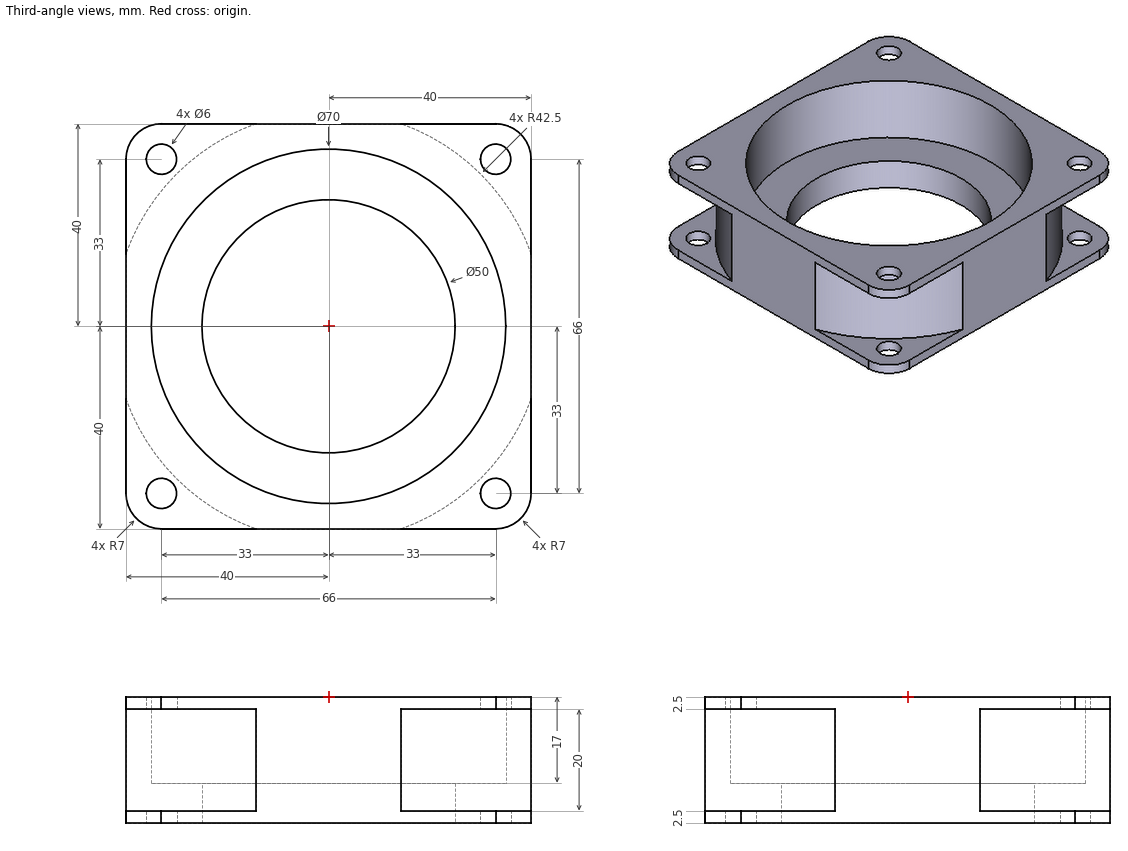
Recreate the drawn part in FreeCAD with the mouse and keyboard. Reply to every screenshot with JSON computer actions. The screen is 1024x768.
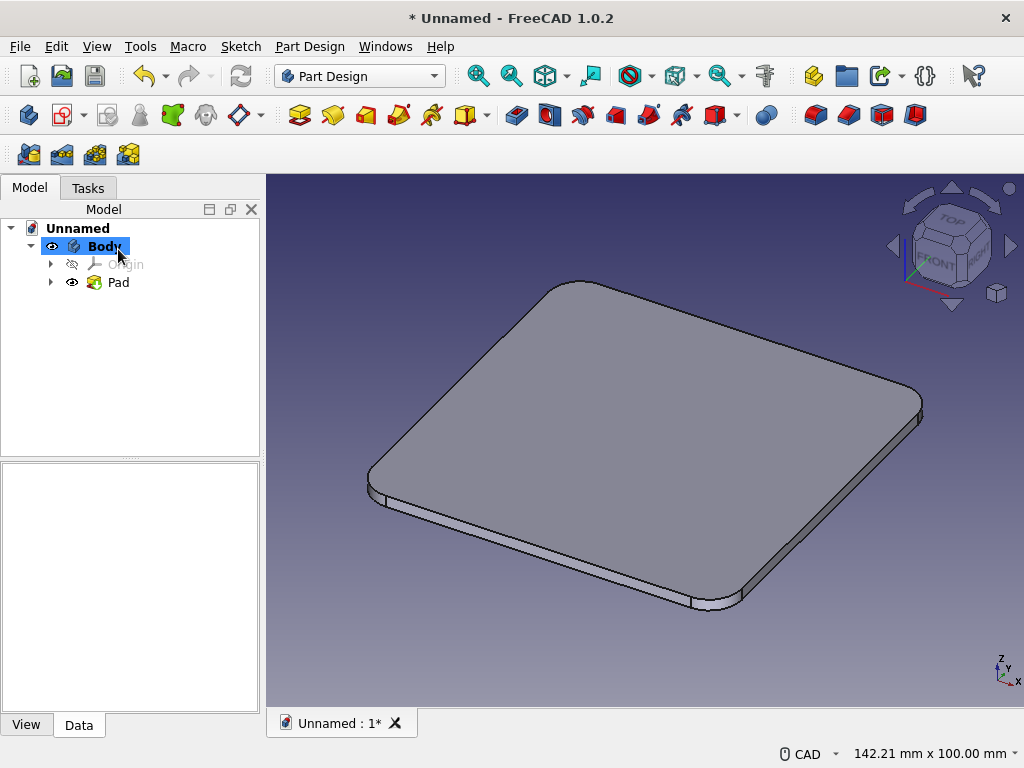
{"action": "key", "text": "5"}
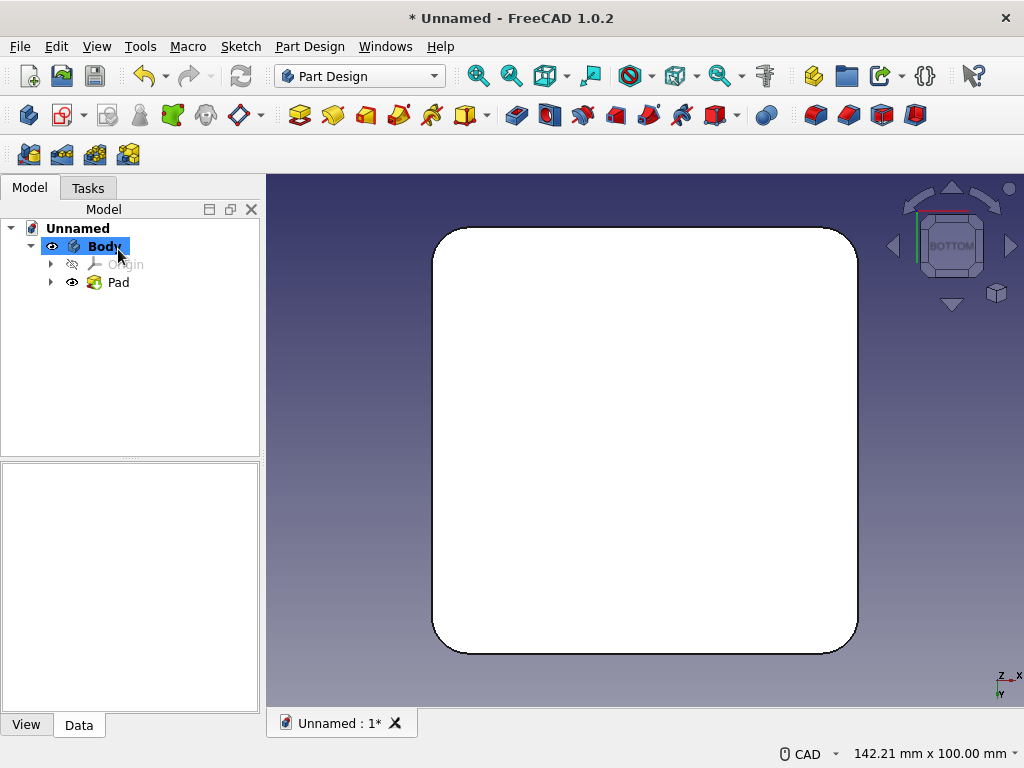
{"action": "left_click", "coordinate": [645, 439]}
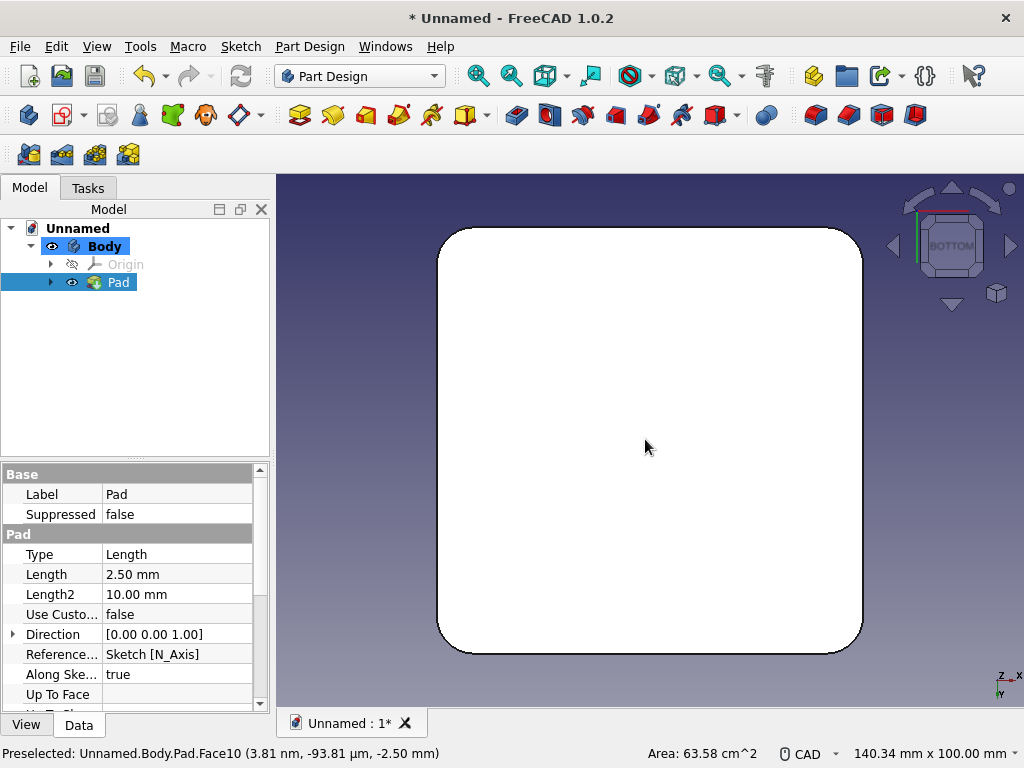
{"action": "left_click", "coordinate": [62, 116]}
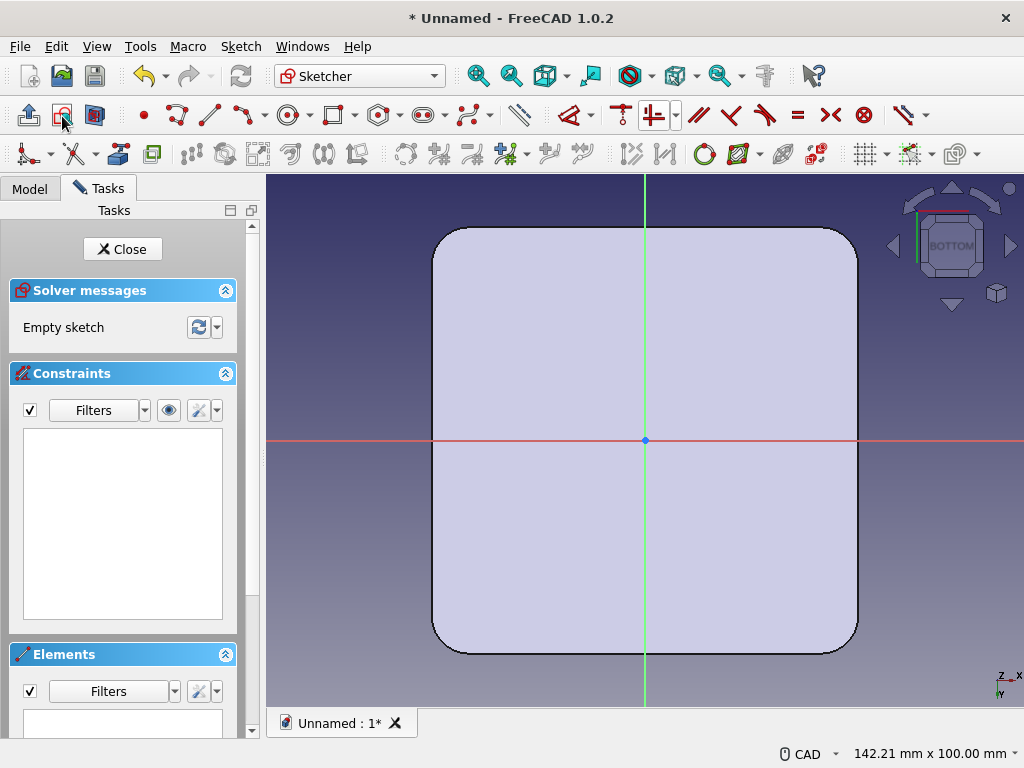
{"action": "scroll", "coordinate": [294, 440], "scroll_direction": "down", "scroll_amount": 1}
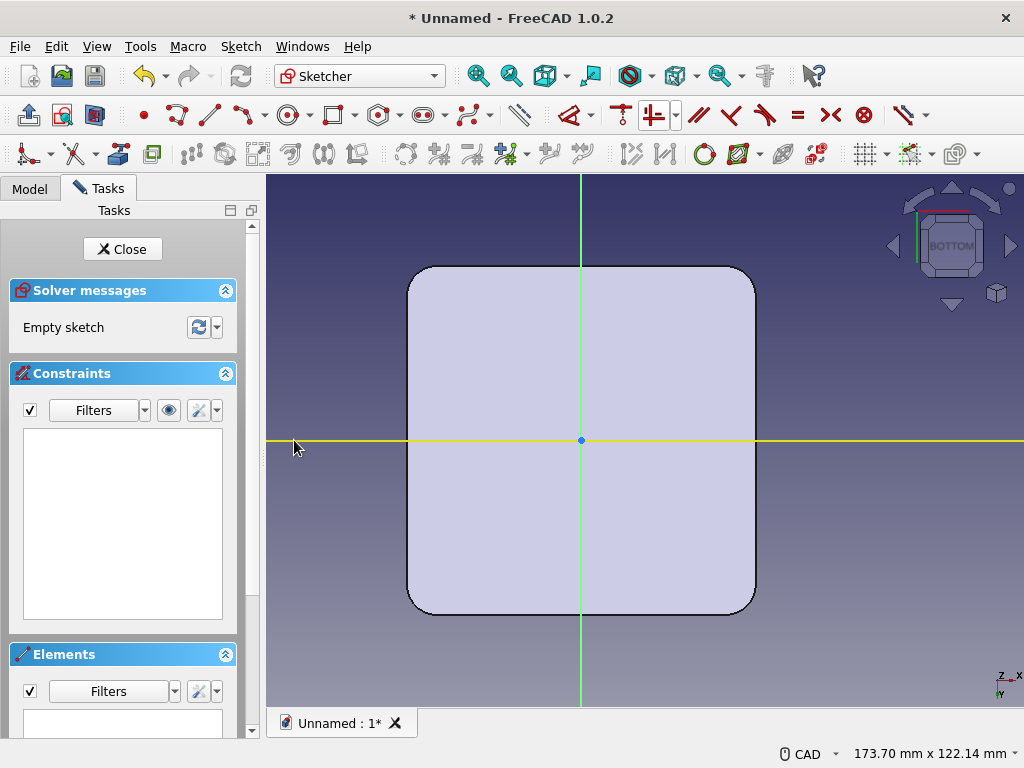
{"action": "left_click", "coordinate": [210, 116]}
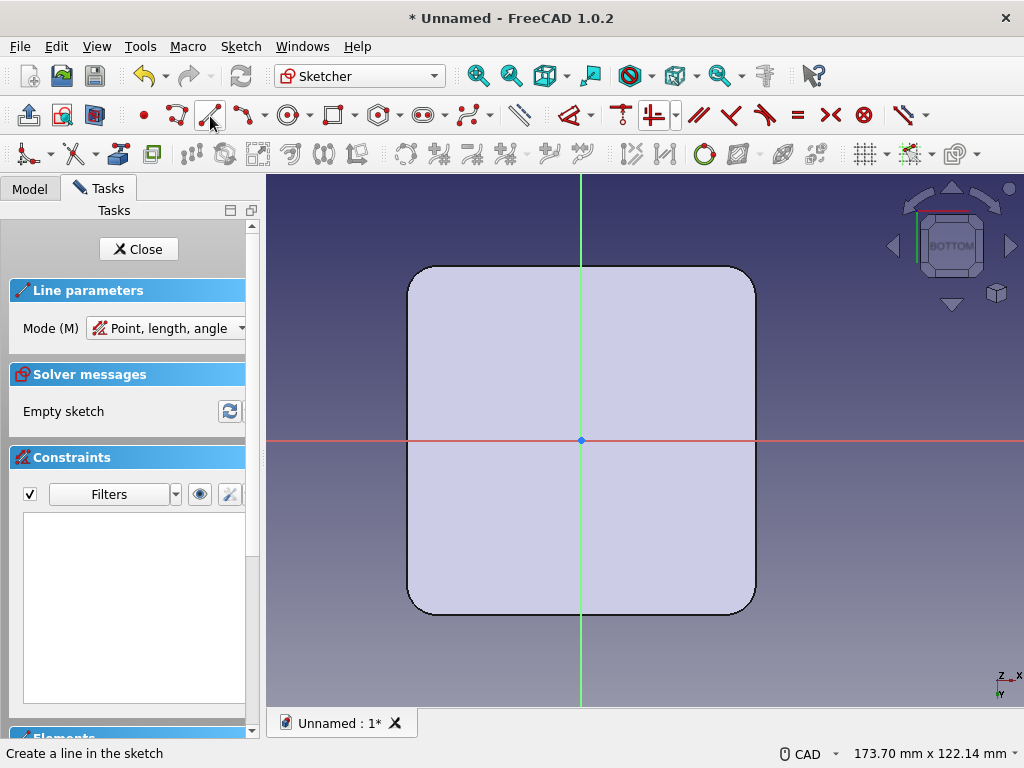
{"action": "left_click", "coordinate": [519, 615]}
{"action": "left_click", "coordinate": [644, 615]}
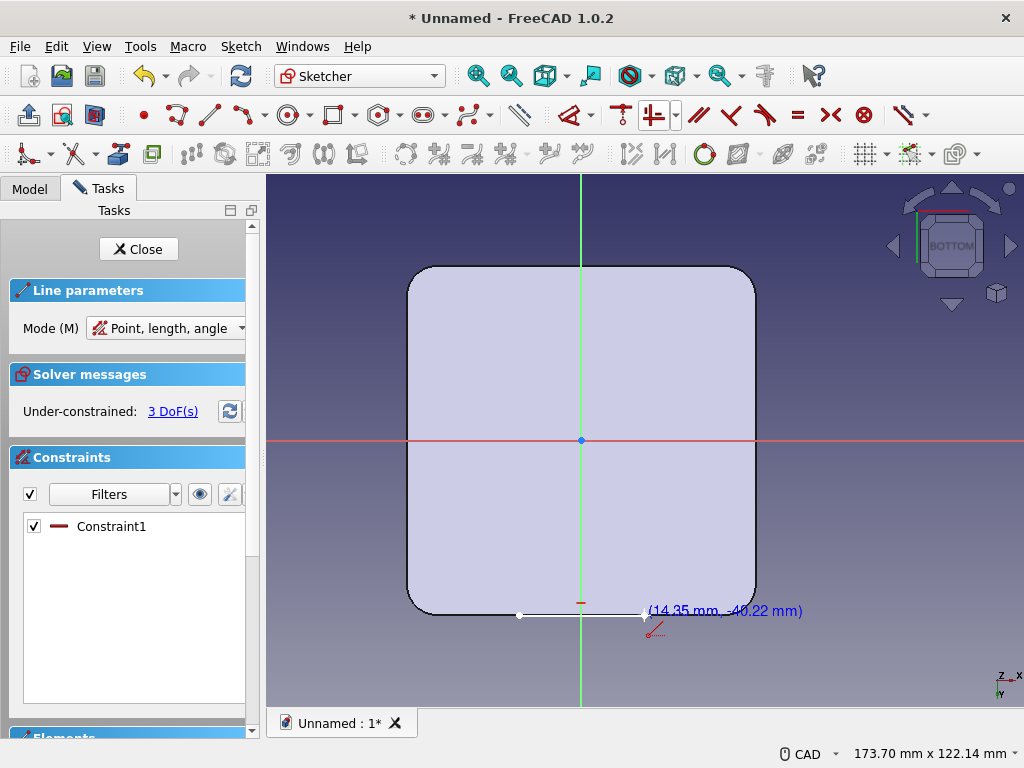
{"action": "left_click", "coordinate": [756, 503]}
{"action": "left_click", "coordinate": [756, 378]}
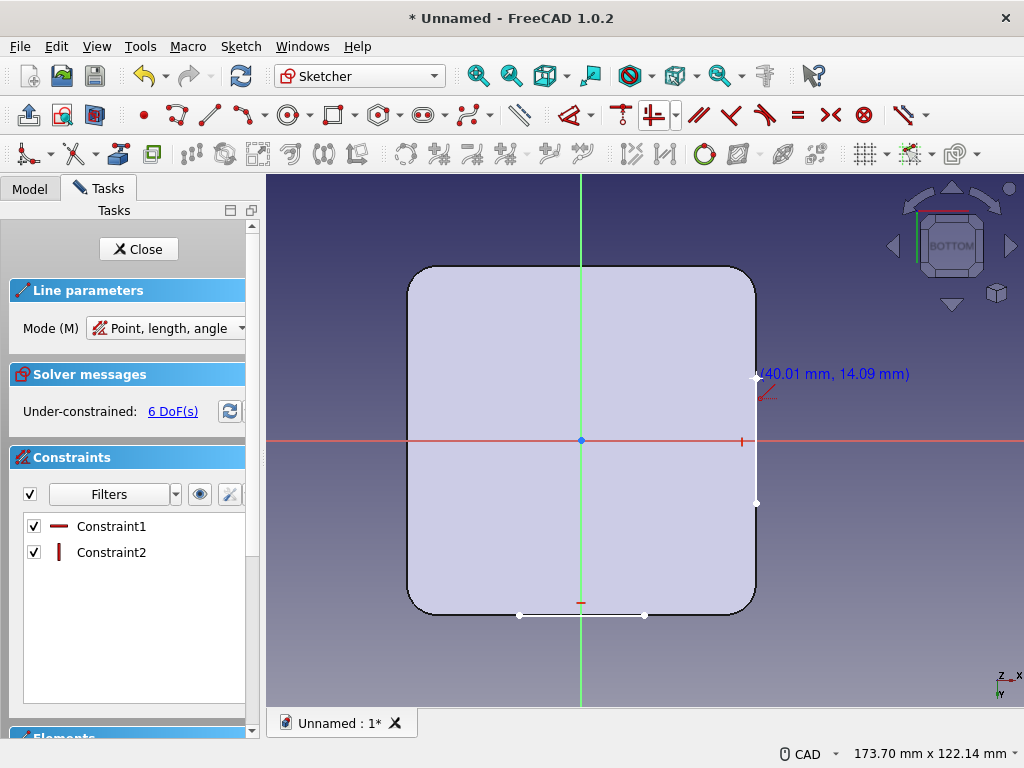
{"action": "left_click", "coordinate": [644, 266]}
{"action": "left_click", "coordinate": [519, 266]}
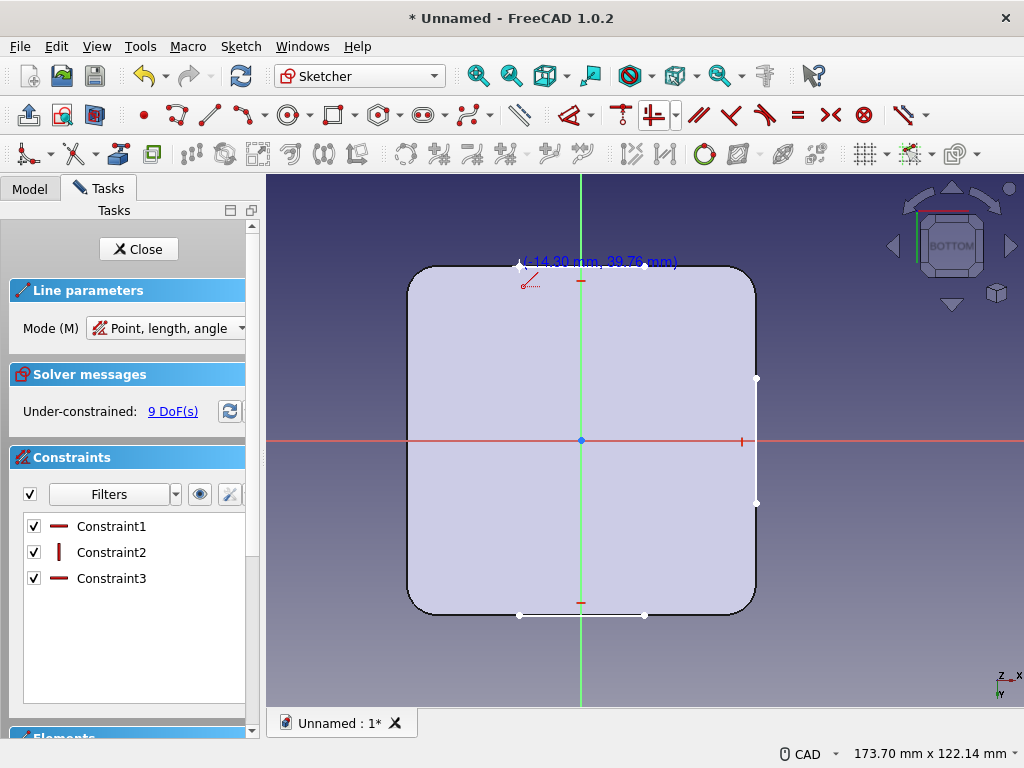
{"action": "left_click", "coordinate": [407, 378]}
{"action": "left_click", "coordinate": [407, 503]}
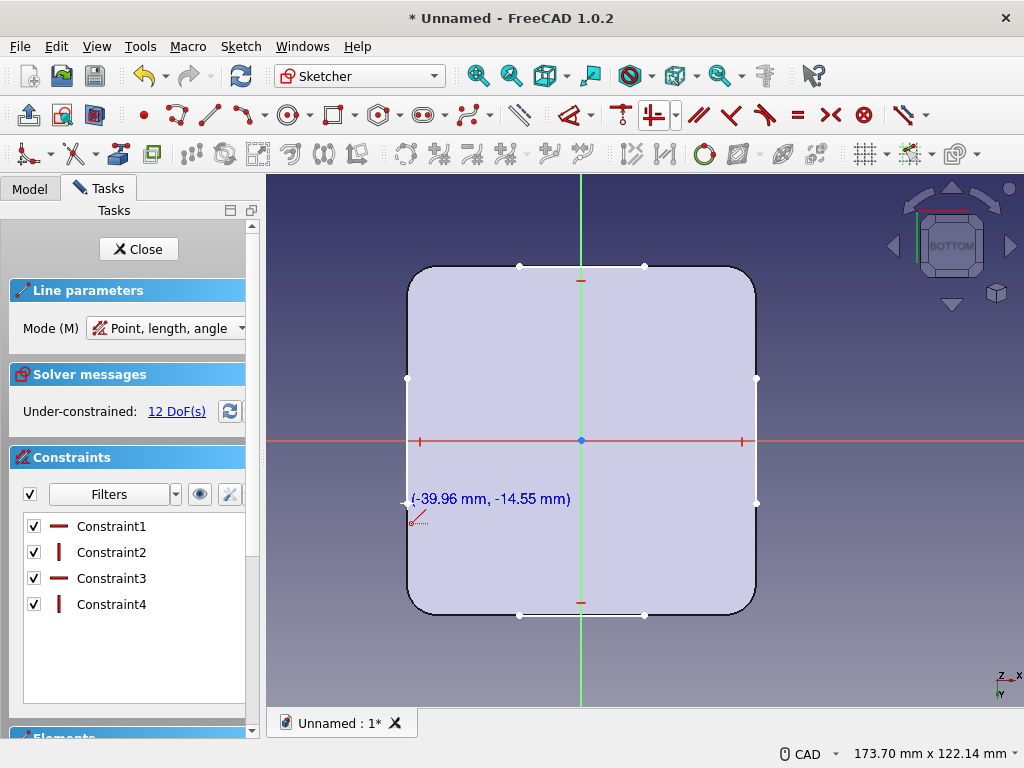
{"action": "left_click", "coordinate": [242, 116]}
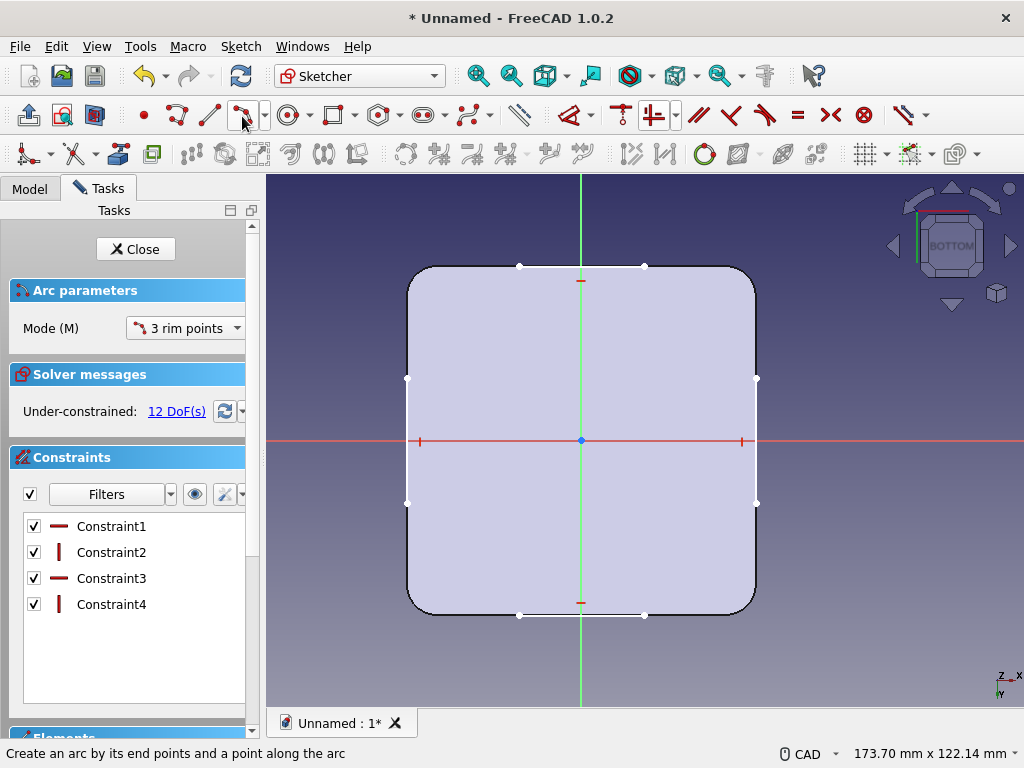
{"action": "left_click", "coordinate": [644, 616]}
{"action": "left_click", "coordinate": [756, 504]}
{"action": "left_click", "coordinate": [713, 572]}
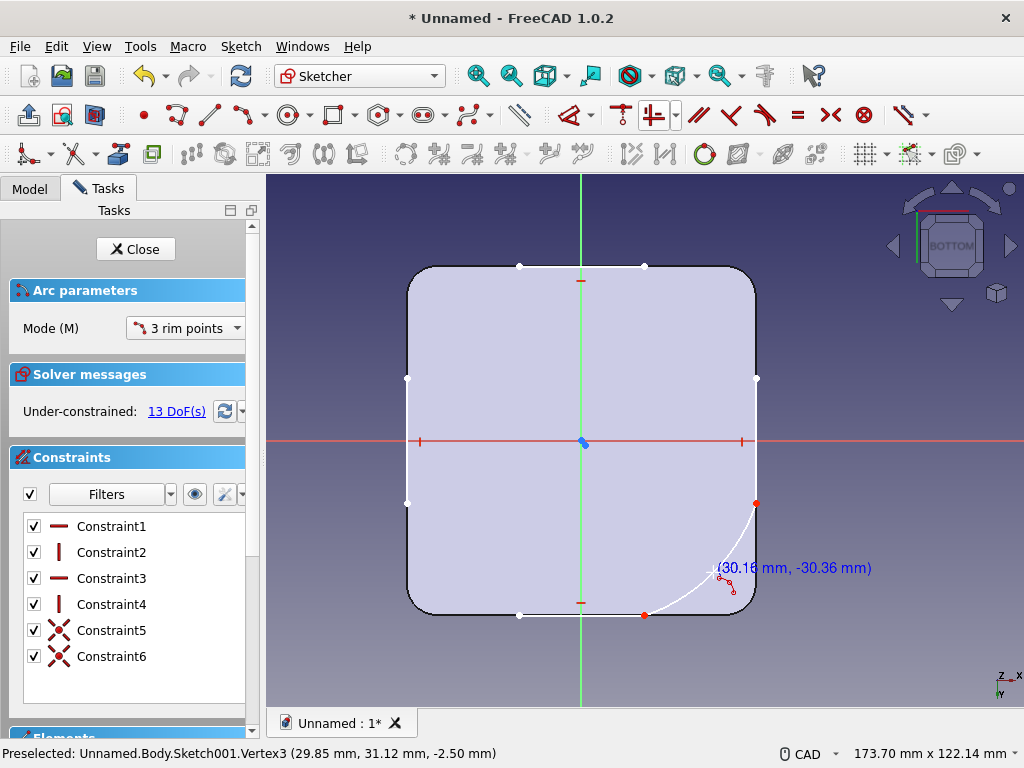
{"action": "left_click", "coordinate": [756, 379]}
{"action": "left_click", "coordinate": [644, 267]}
{"action": "left_click", "coordinate": [713, 309]}